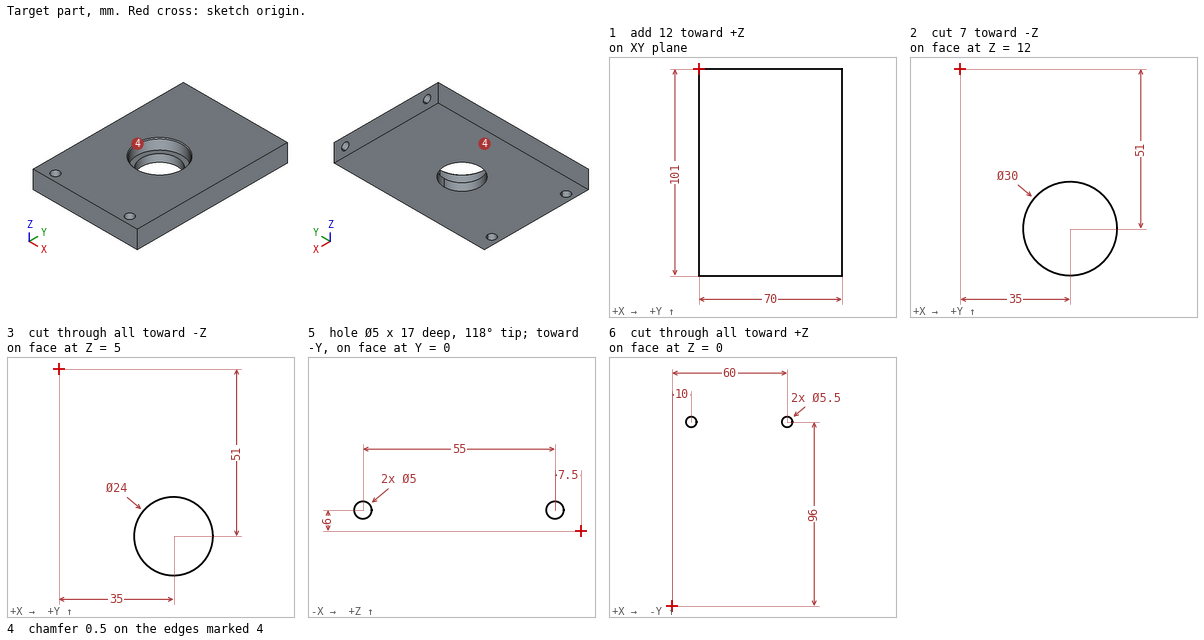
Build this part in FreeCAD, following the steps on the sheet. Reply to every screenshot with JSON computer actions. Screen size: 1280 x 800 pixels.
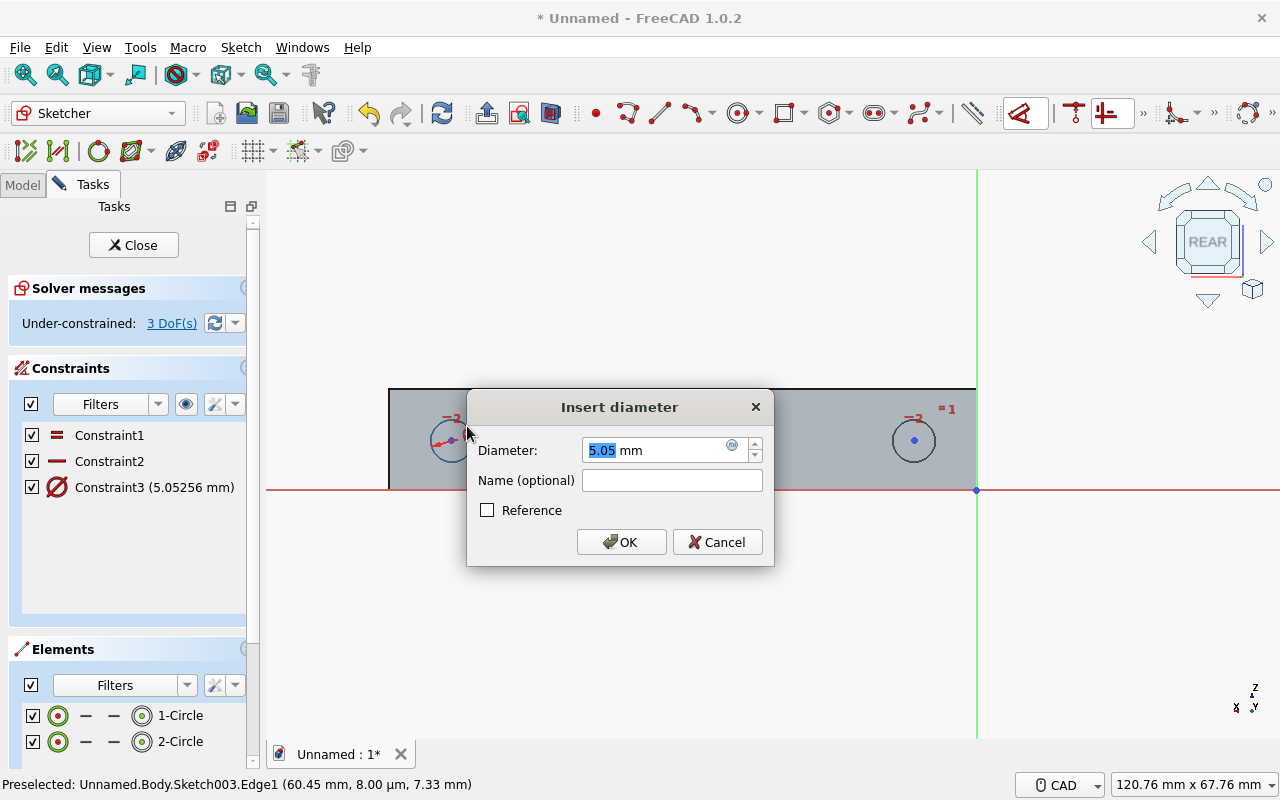
{"action": "type", "text": "5"}
{"action": "key", "text": "Return"}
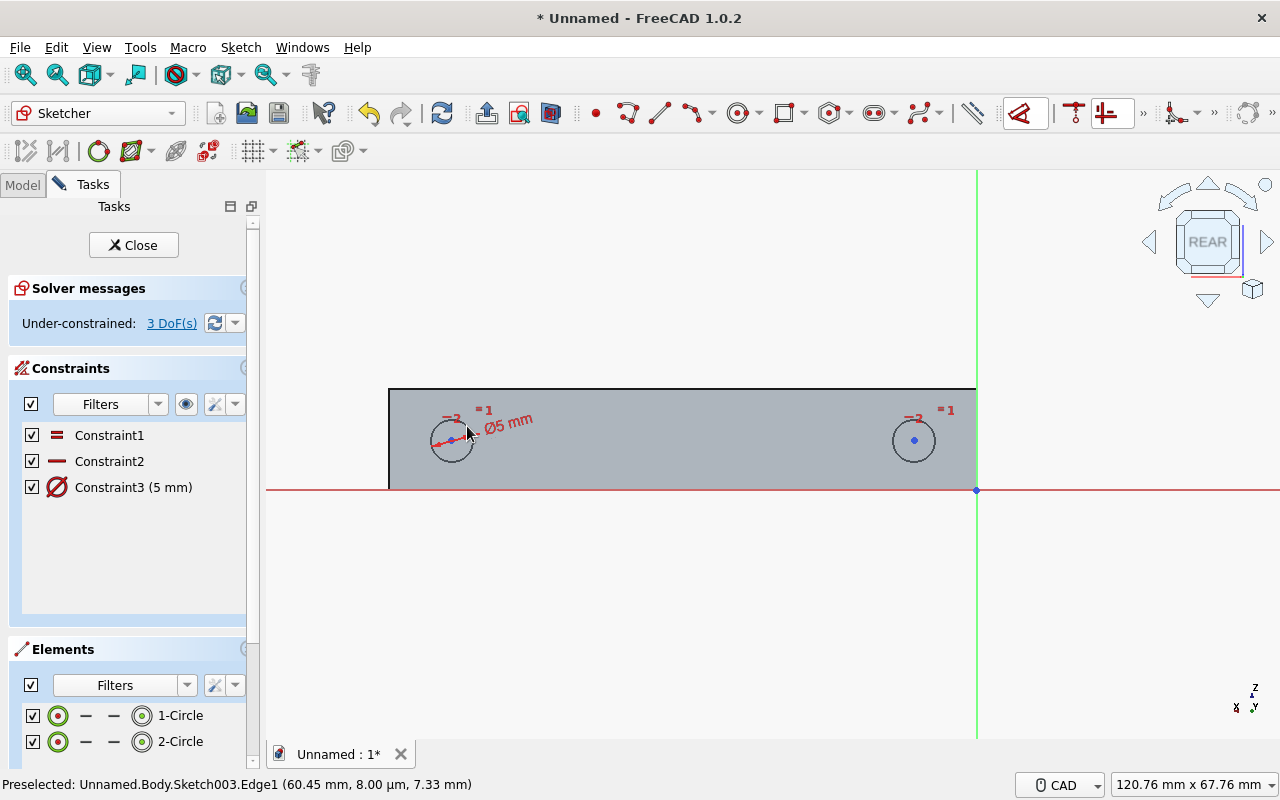
{"action": "left_click", "coordinate": [452, 441]}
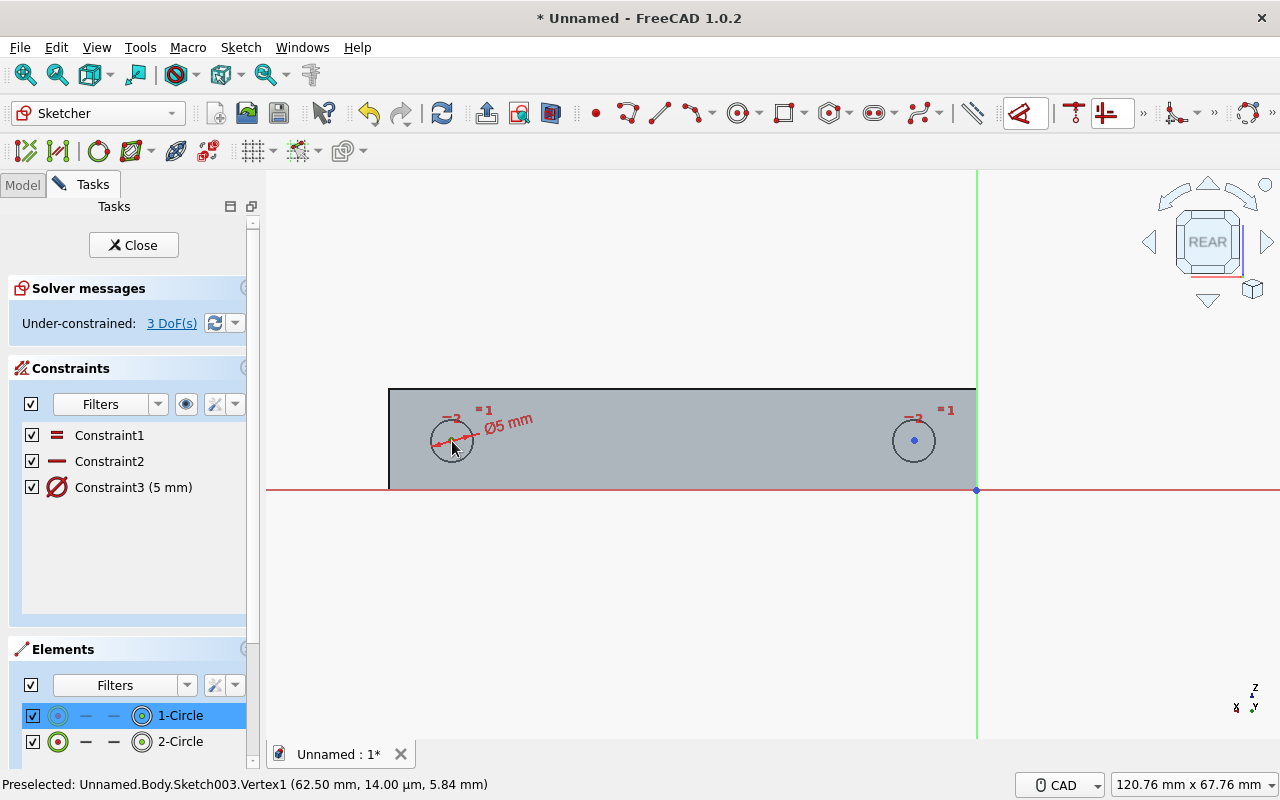
{"action": "left_click", "coordinate": [1042, 114]}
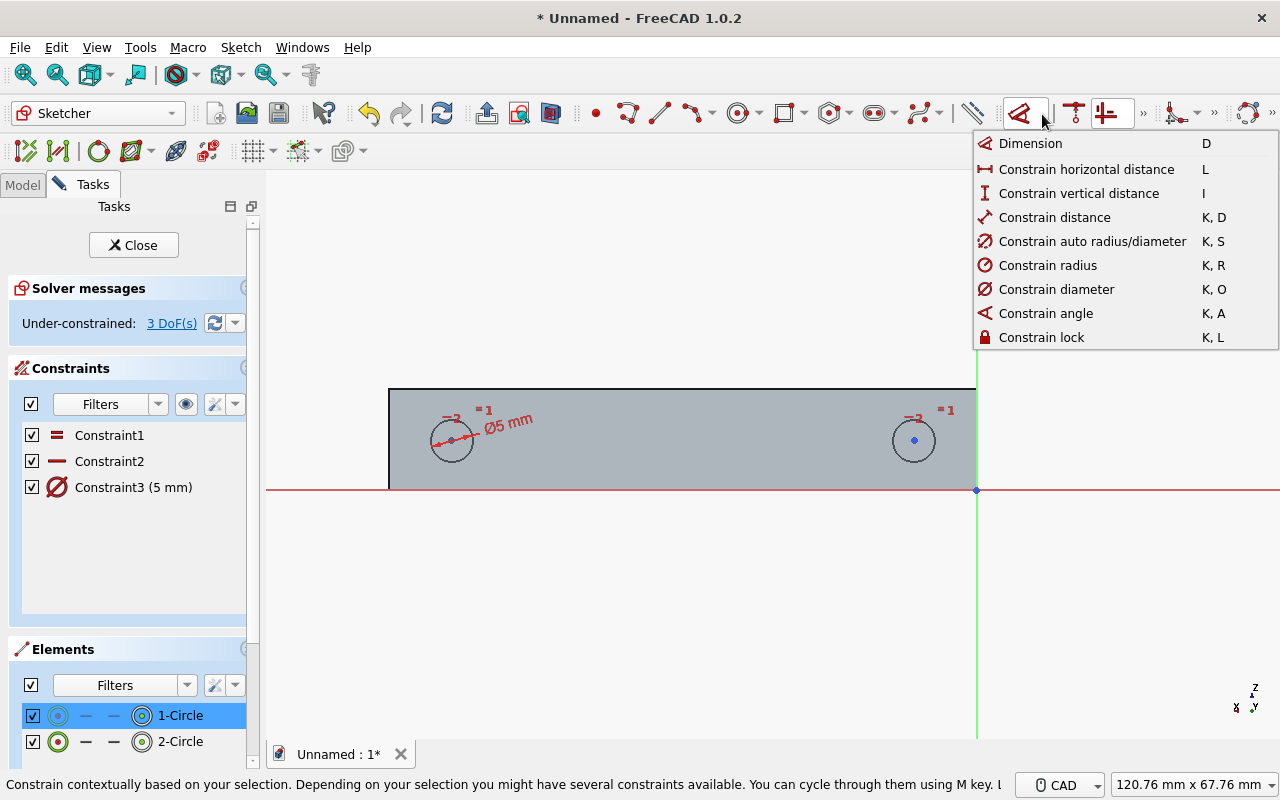
{"action": "left_click", "coordinate": [1126, 193]}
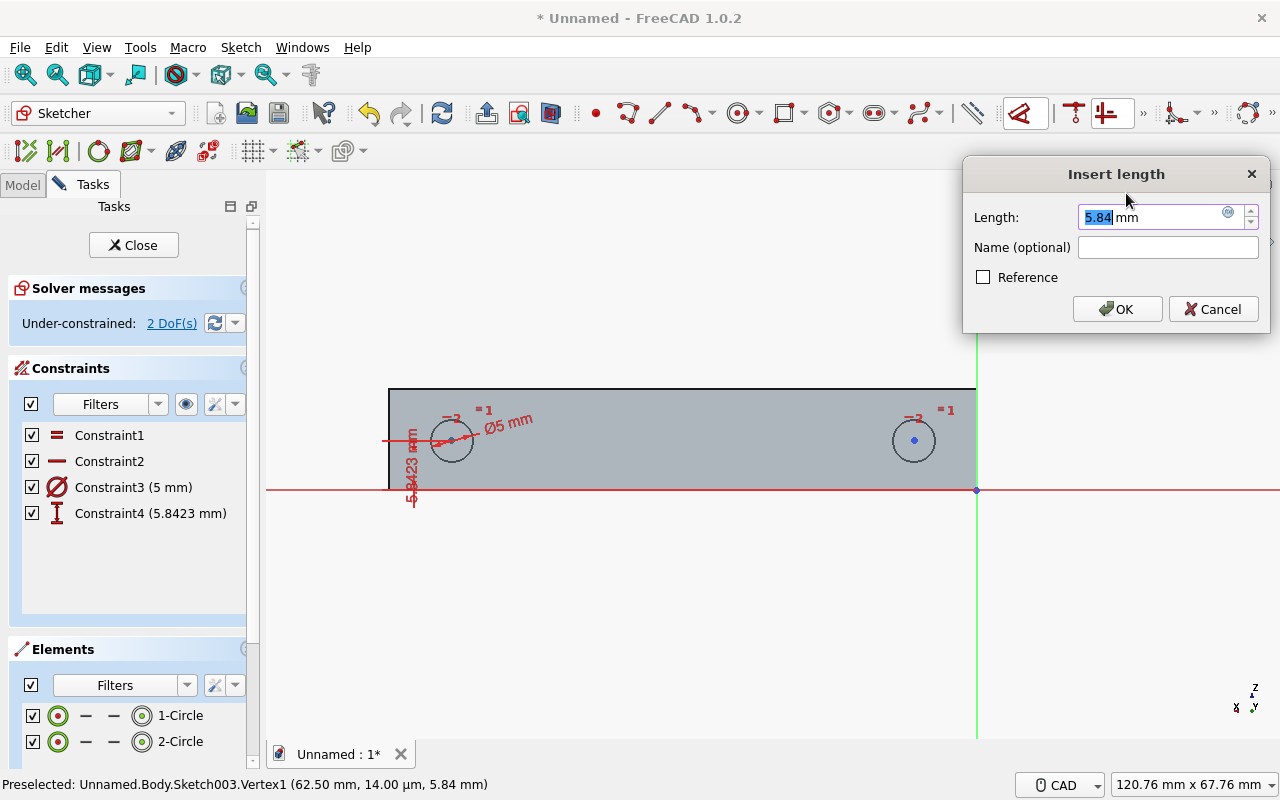
{"action": "type", "text": "6"}
{"action": "key", "text": "Return"}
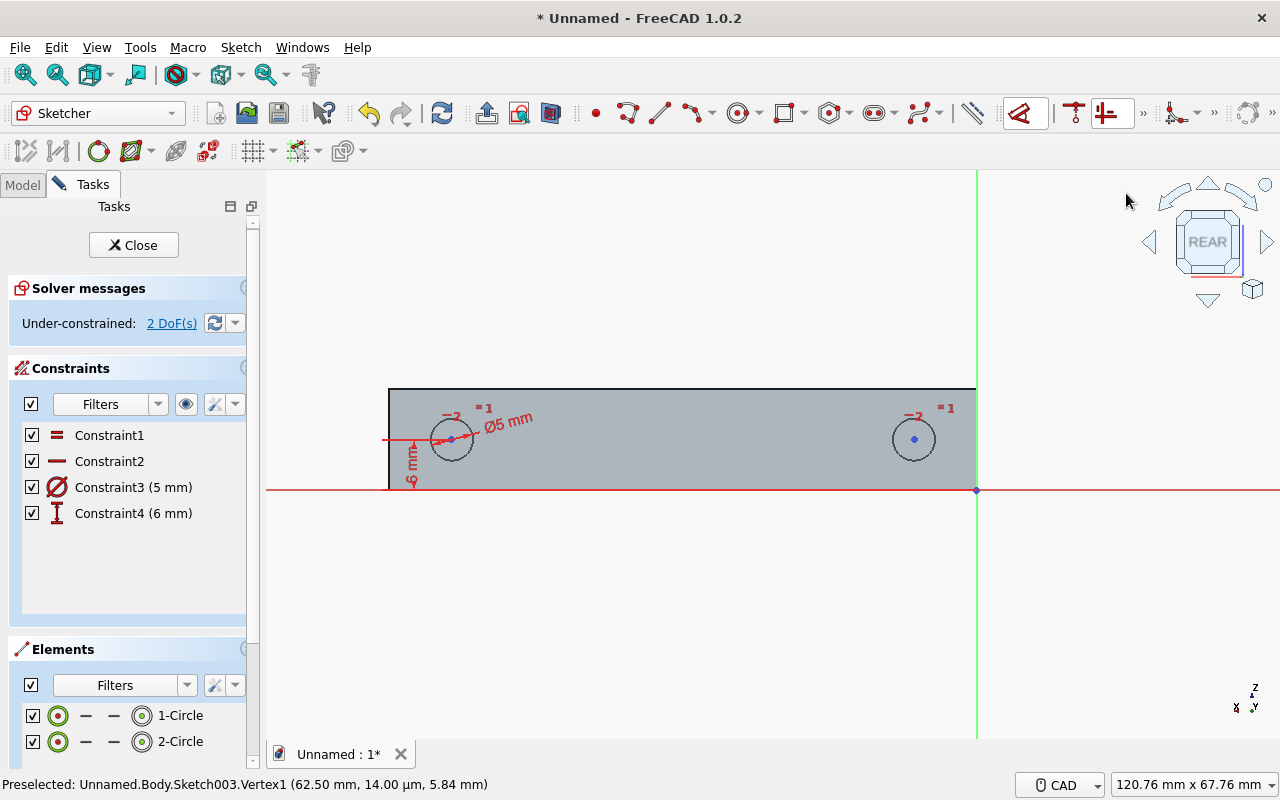
{"action": "left_click", "coordinate": [914, 440]}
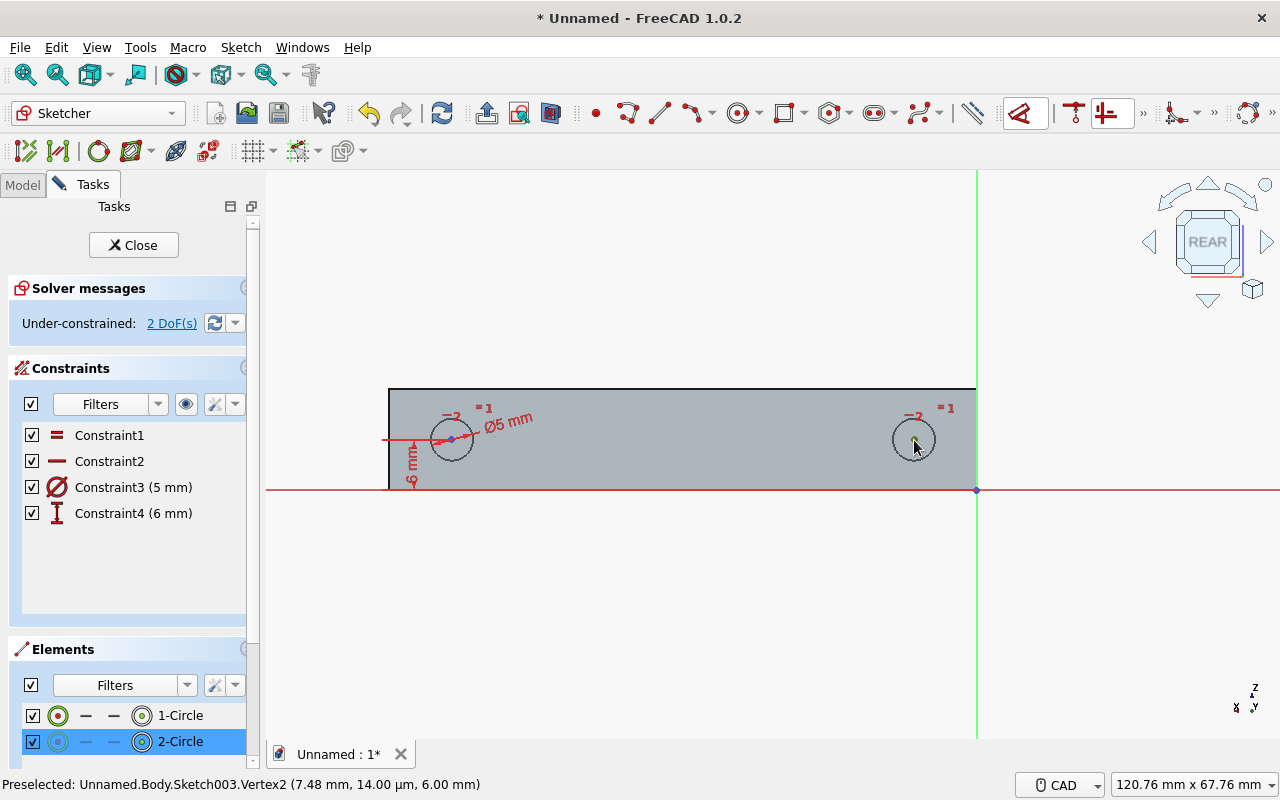
{"action": "key", "text": "l"}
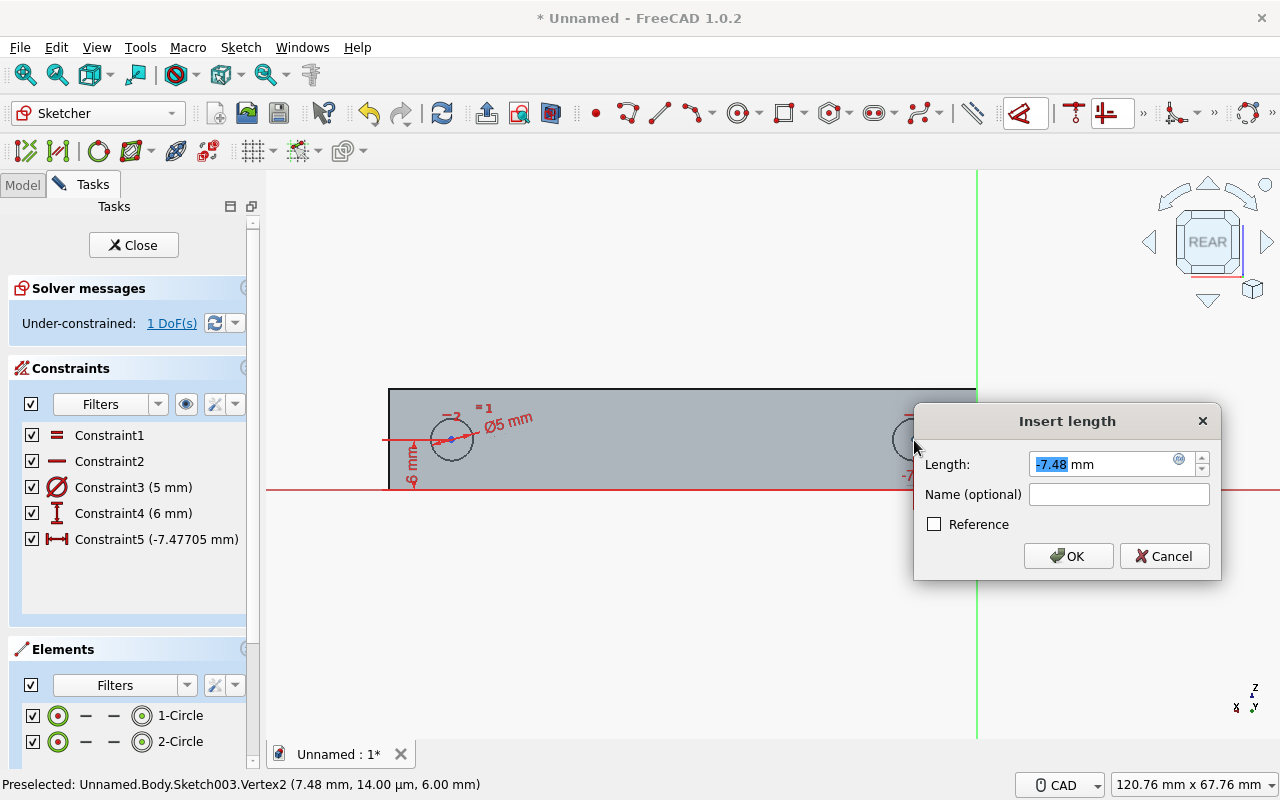
{"action": "type", "text": "-7.5"}
{"action": "key", "text": "Return"}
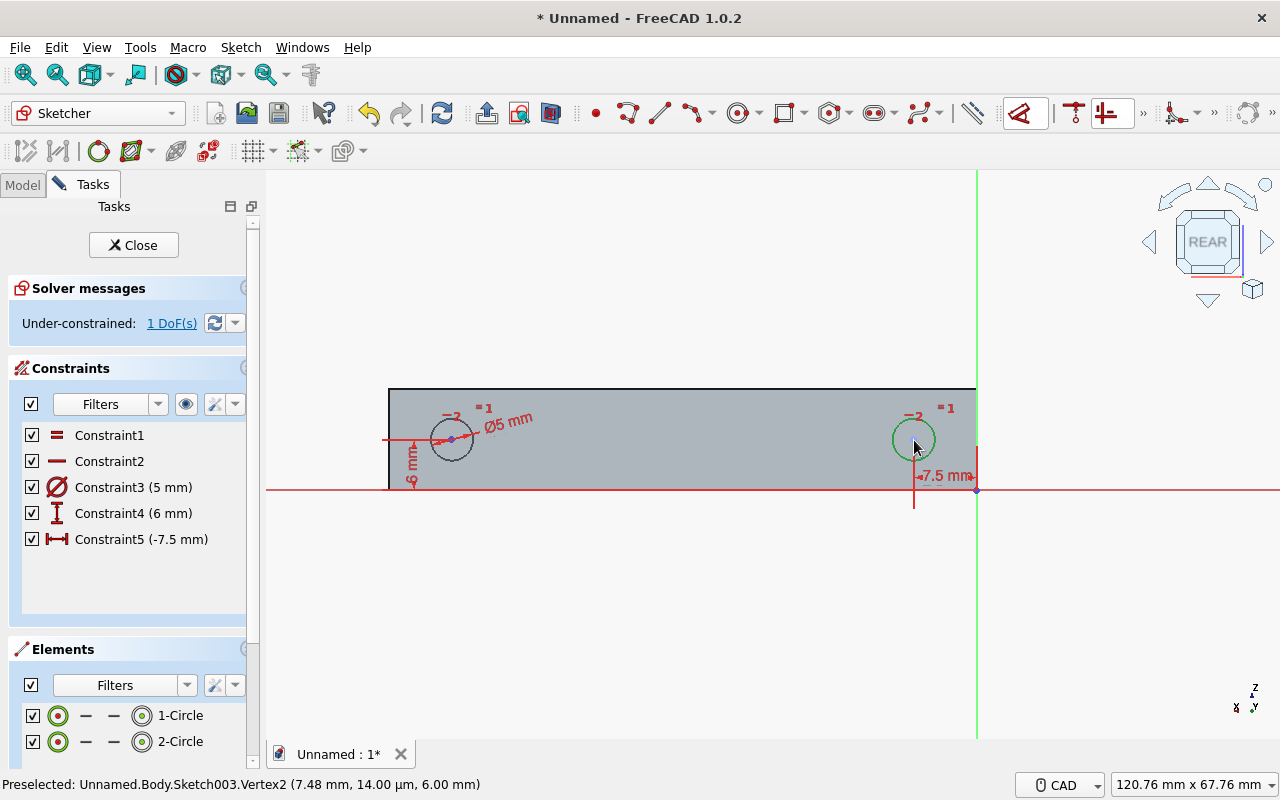
{"action": "left_click", "coordinate": [452, 440]}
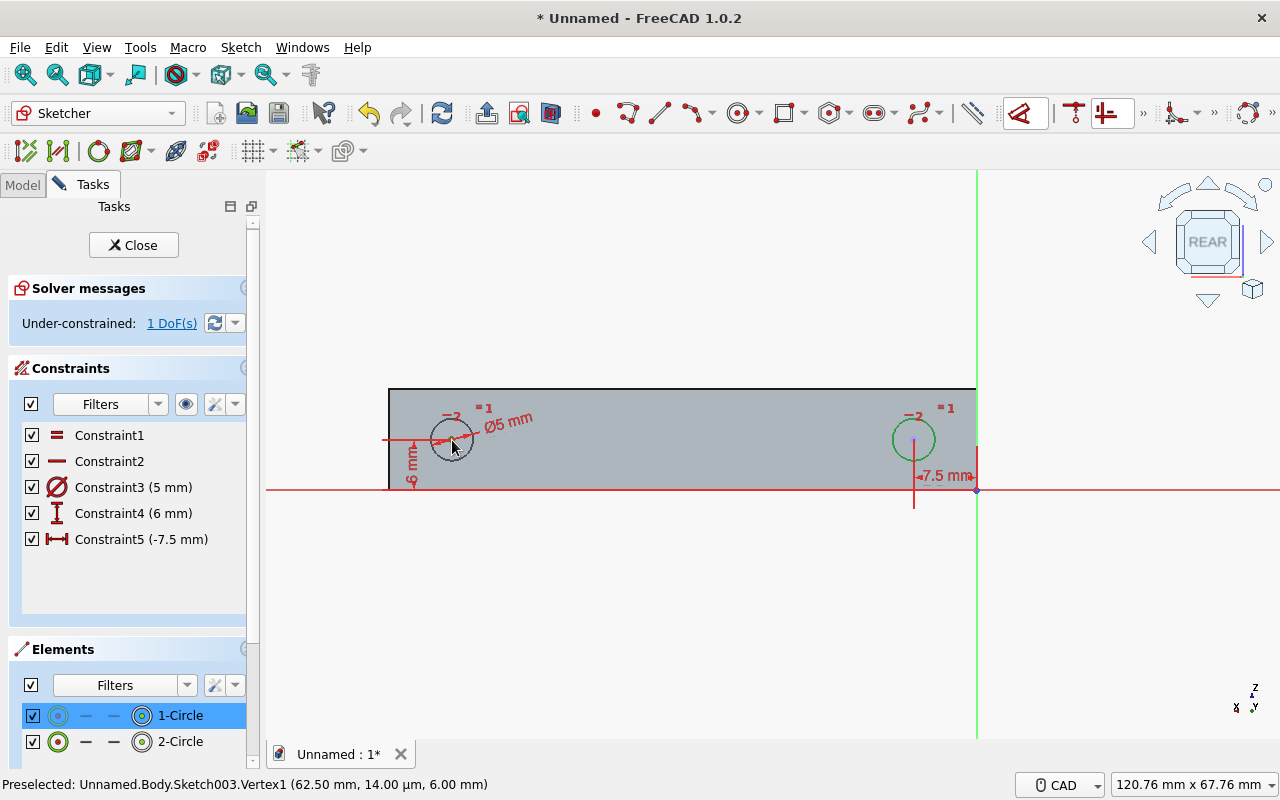
{"action": "left_click", "coordinate": [914, 440]}